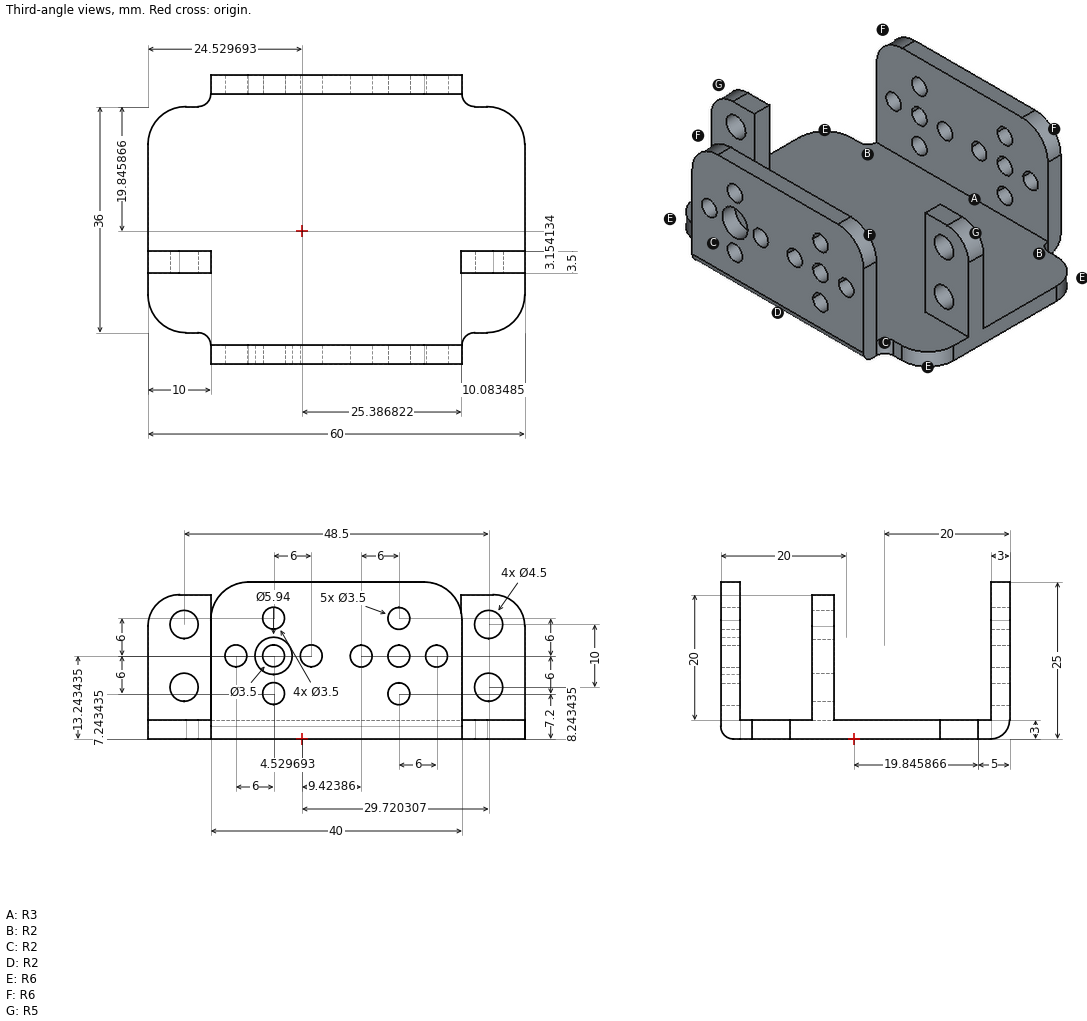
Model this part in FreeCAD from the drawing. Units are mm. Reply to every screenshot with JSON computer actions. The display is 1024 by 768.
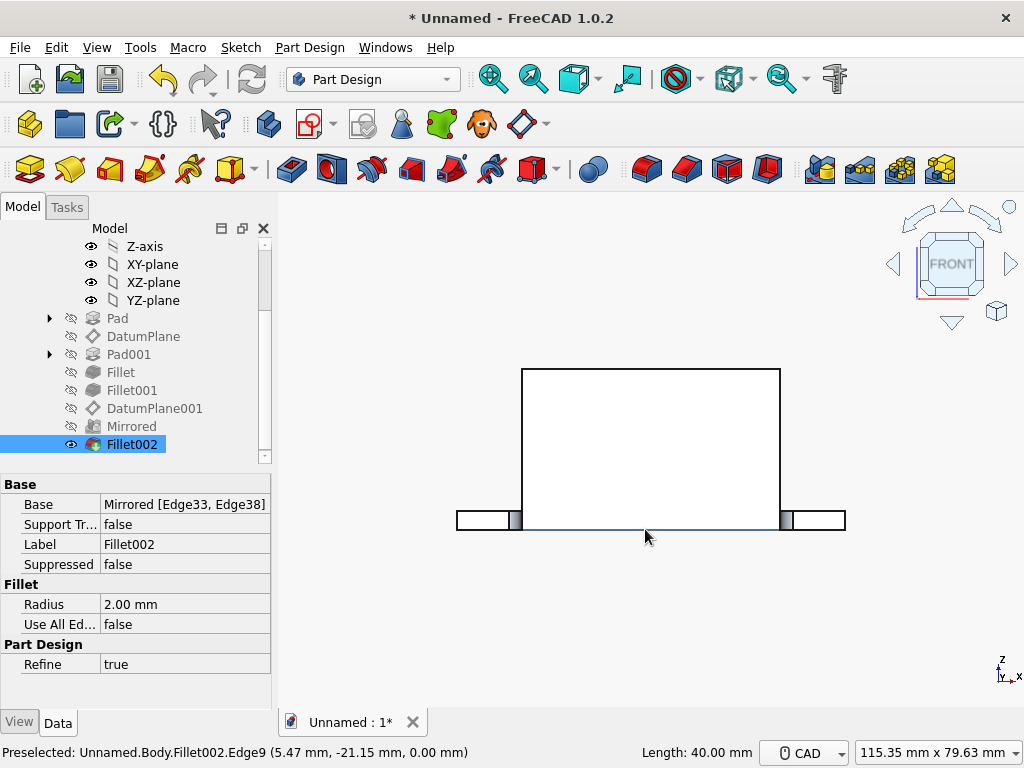
{"action": "left_click", "coordinate": [648, 170]}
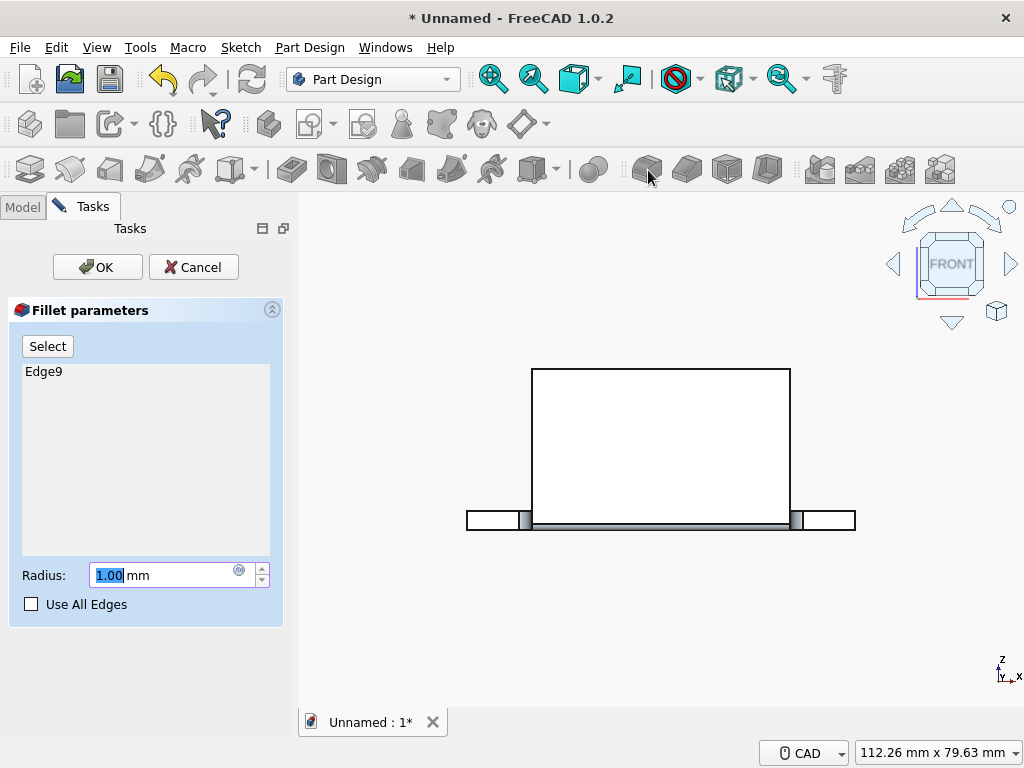
{"action": "type", "text": "2"}
{"action": "key", "text": "Tab"}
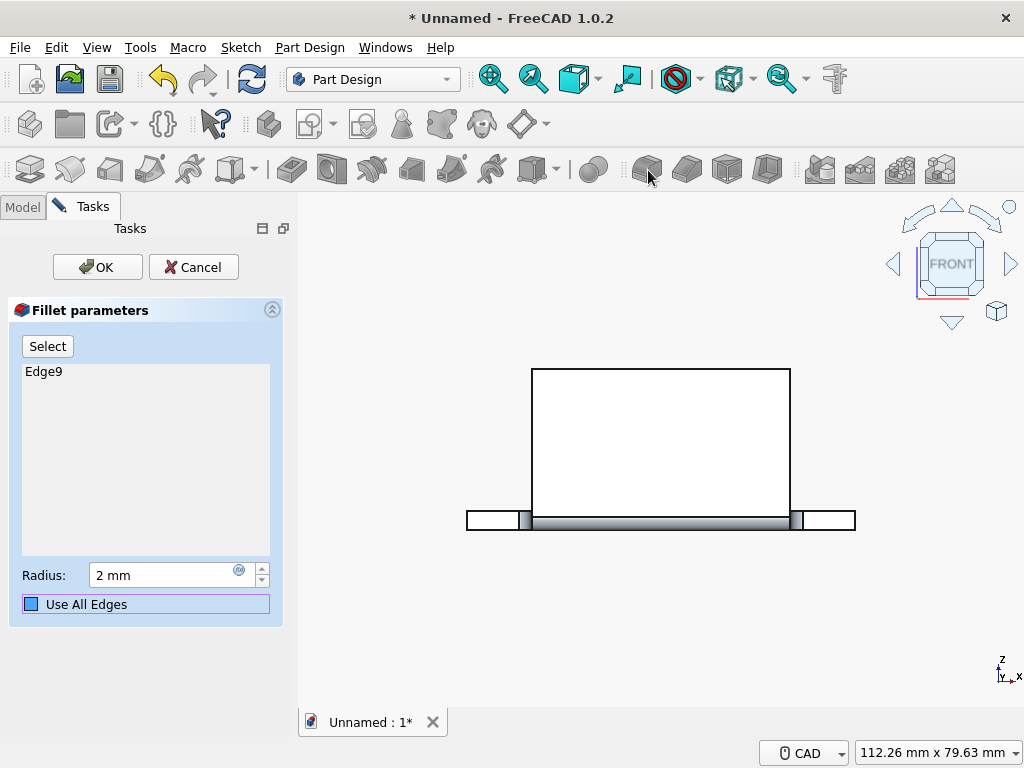
{"action": "left_click", "coordinate": [98, 267]}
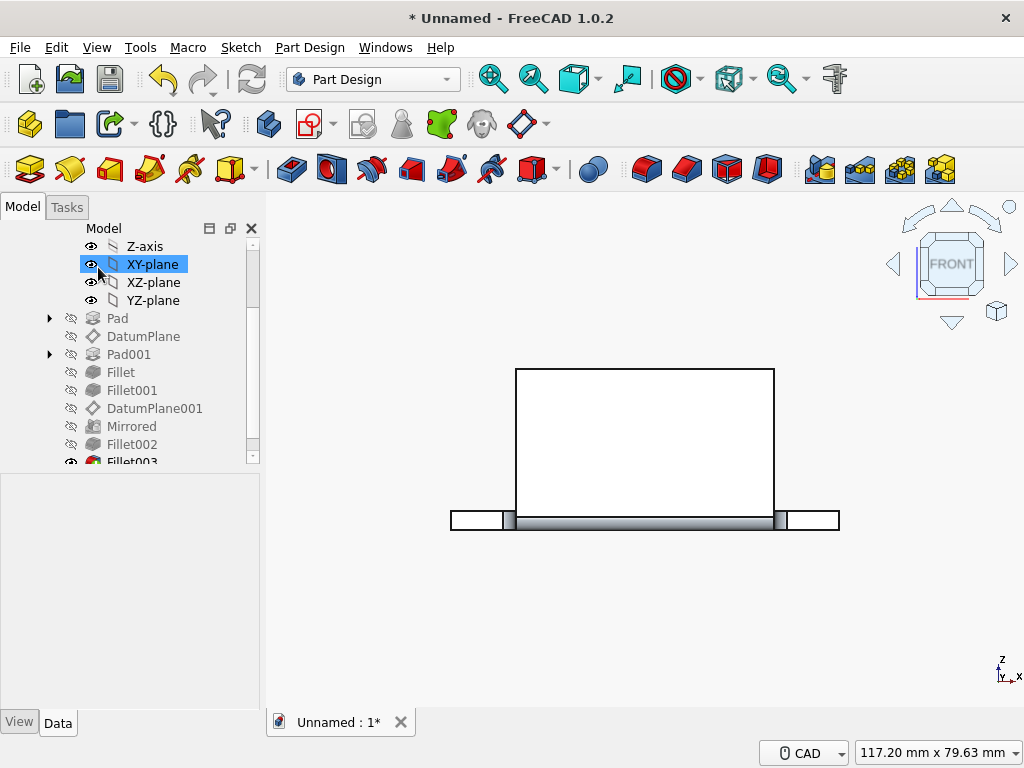
{"action": "left_click", "coordinate": [451, 520]}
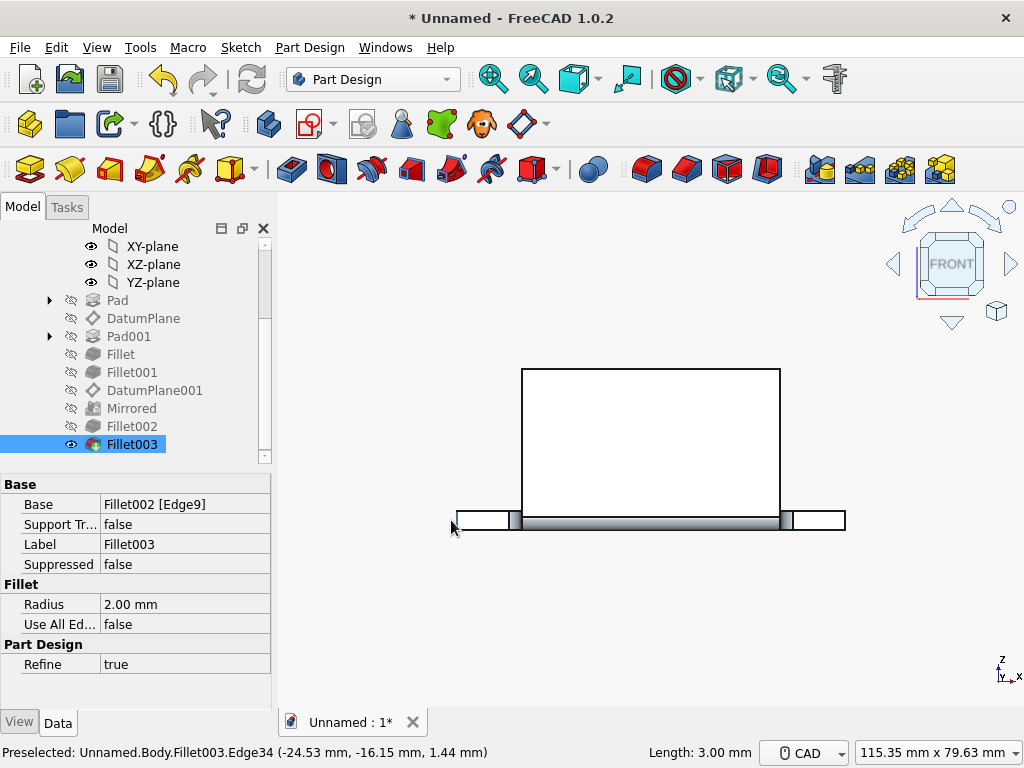
{"action": "left_click", "coordinate": [845, 520], "text": "ctrl"}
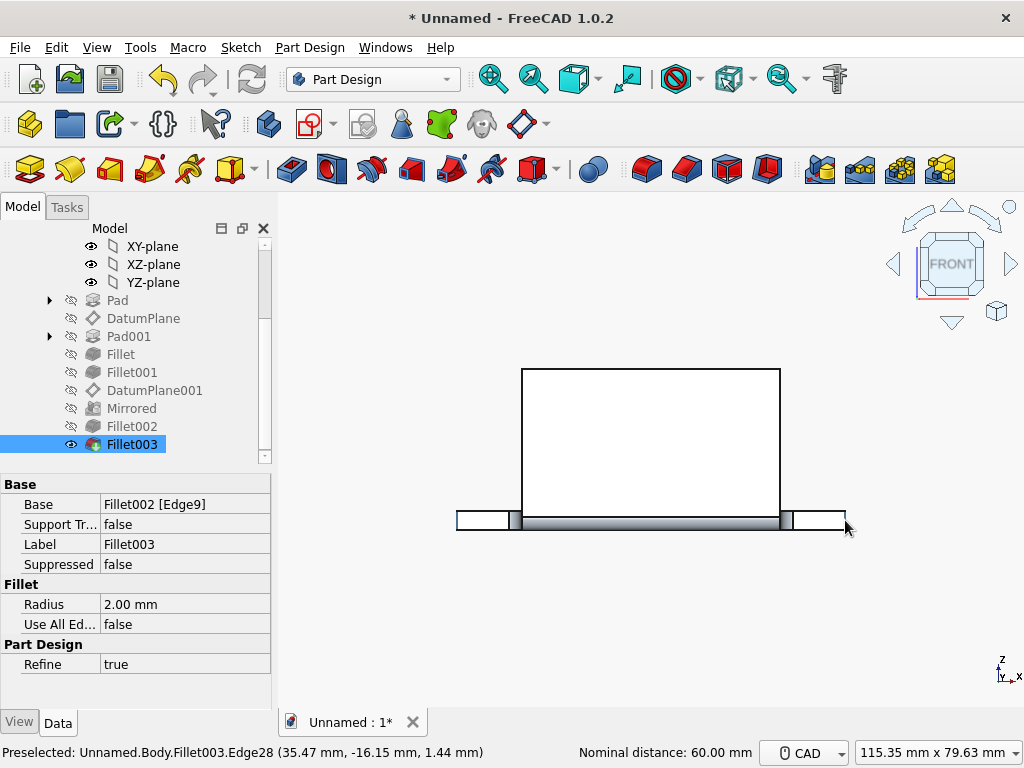
{"action": "scroll", "coordinate": [457, 520], "scroll_direction": "up", "scroll_amount": 4}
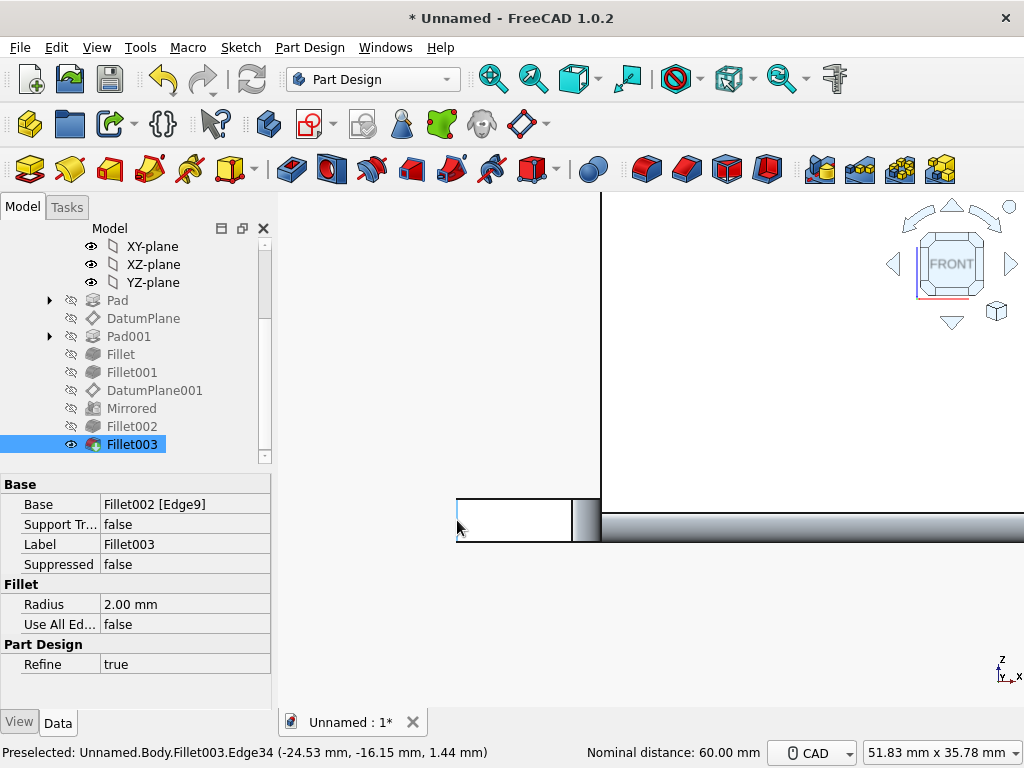
{"action": "left_click", "coordinate": [494, 80]}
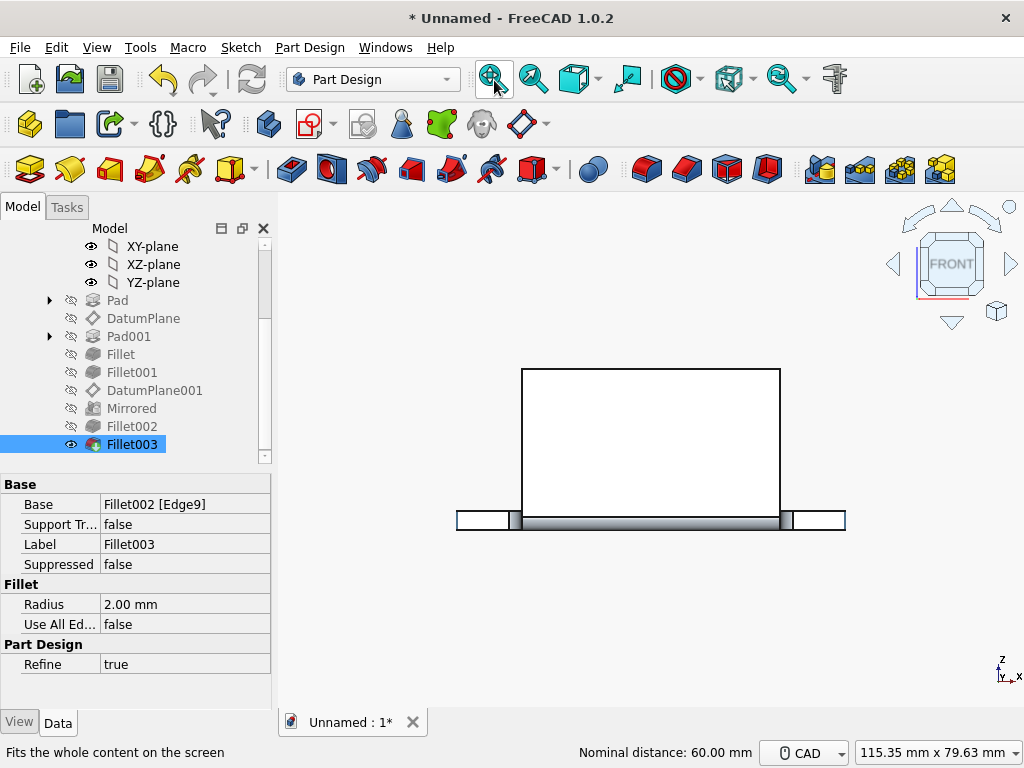
{"action": "key", "text": "0"}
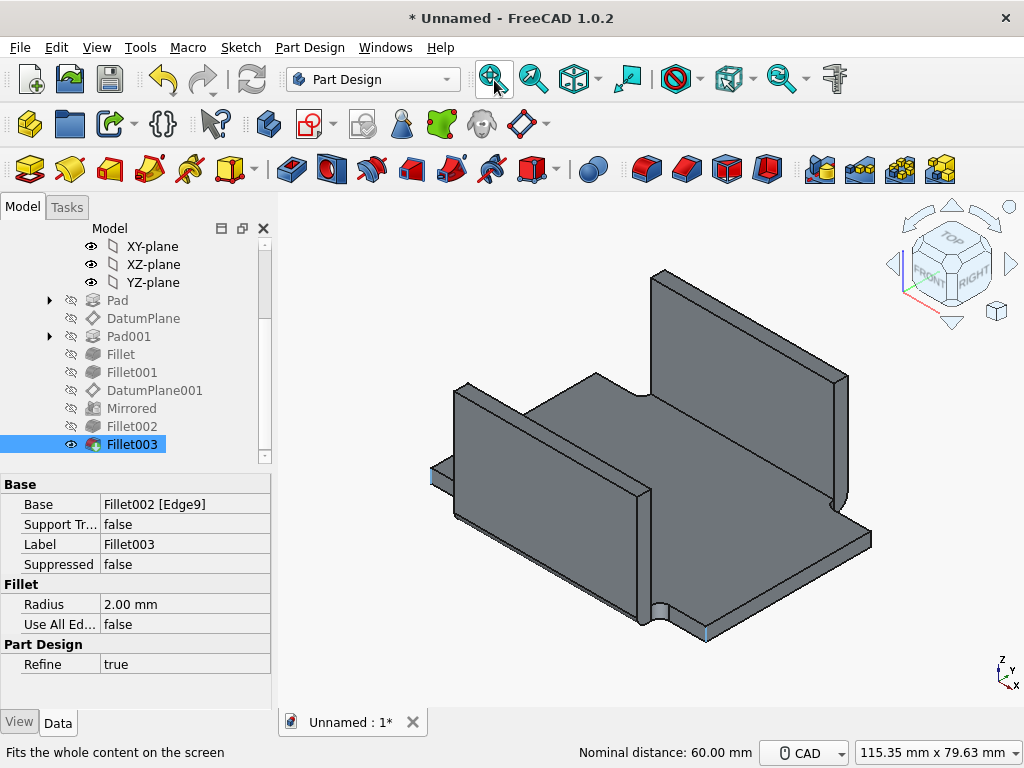
{"action": "scroll", "coordinate": [596, 380], "scroll_direction": "up", "scroll_amount": 4}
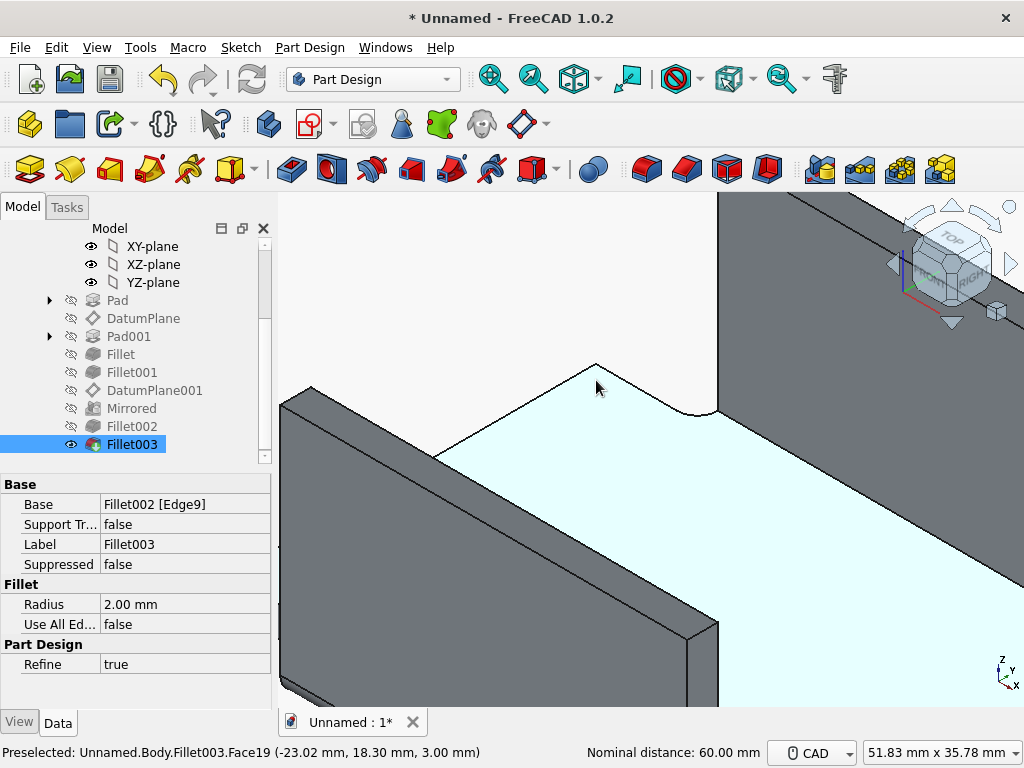
{"action": "left_click", "coordinate": [494, 80]}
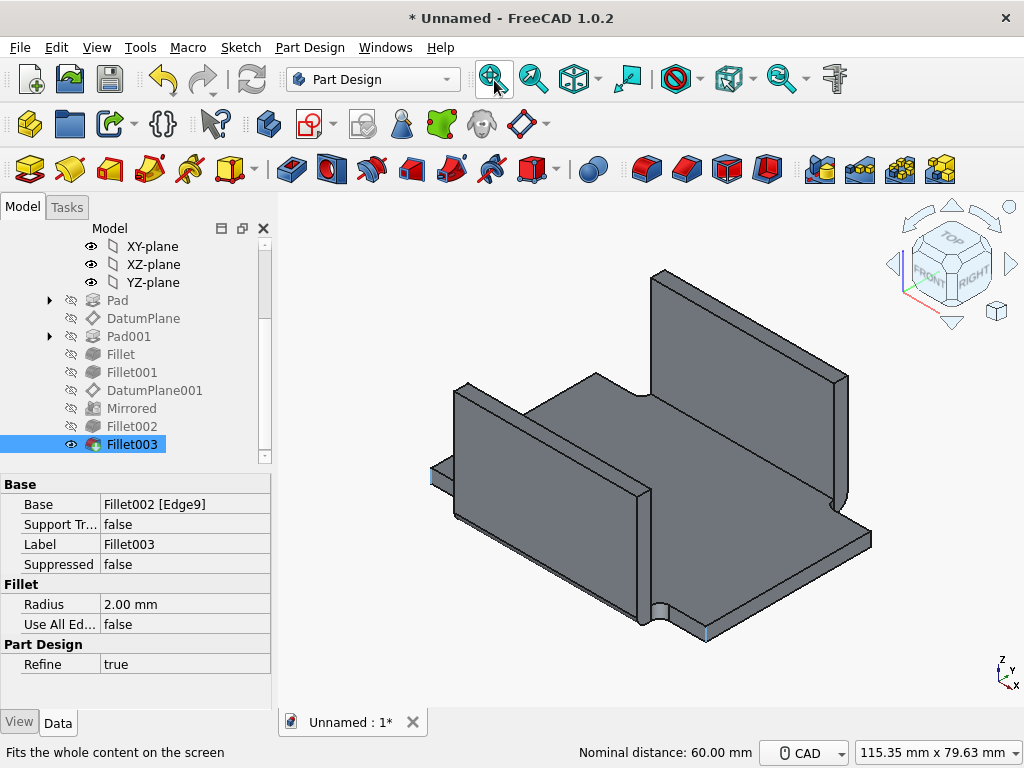
{"action": "key", "text": "2"}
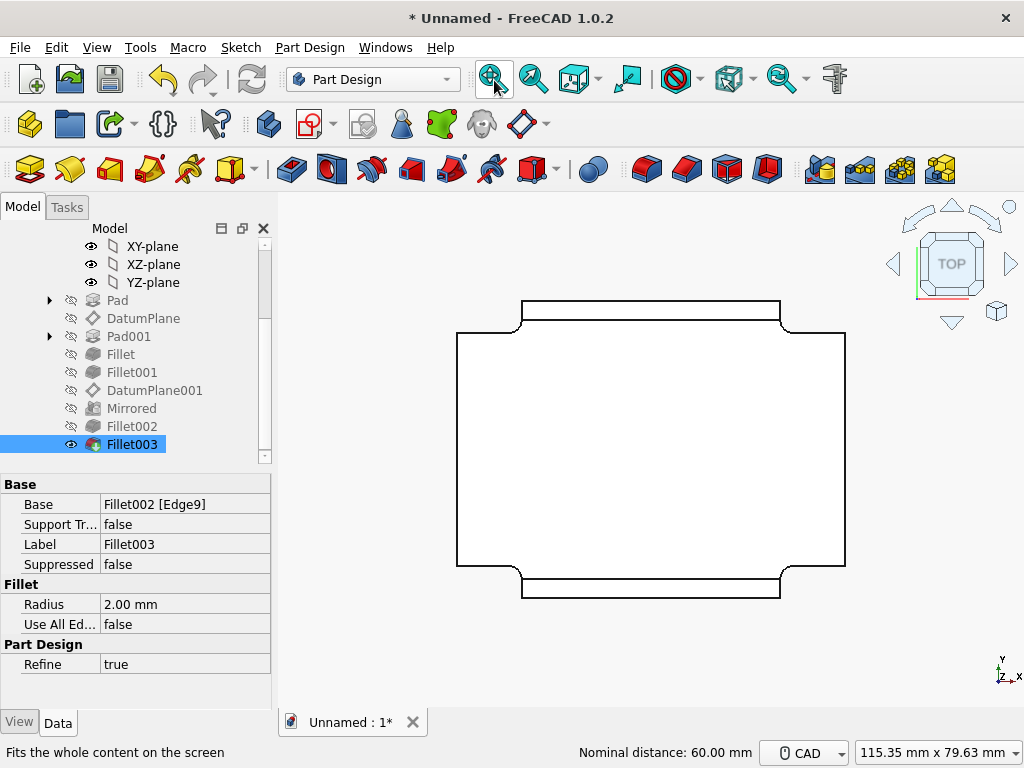
{"action": "scroll", "coordinate": [457, 332], "scroll_direction": "up", "scroll_amount": 4}